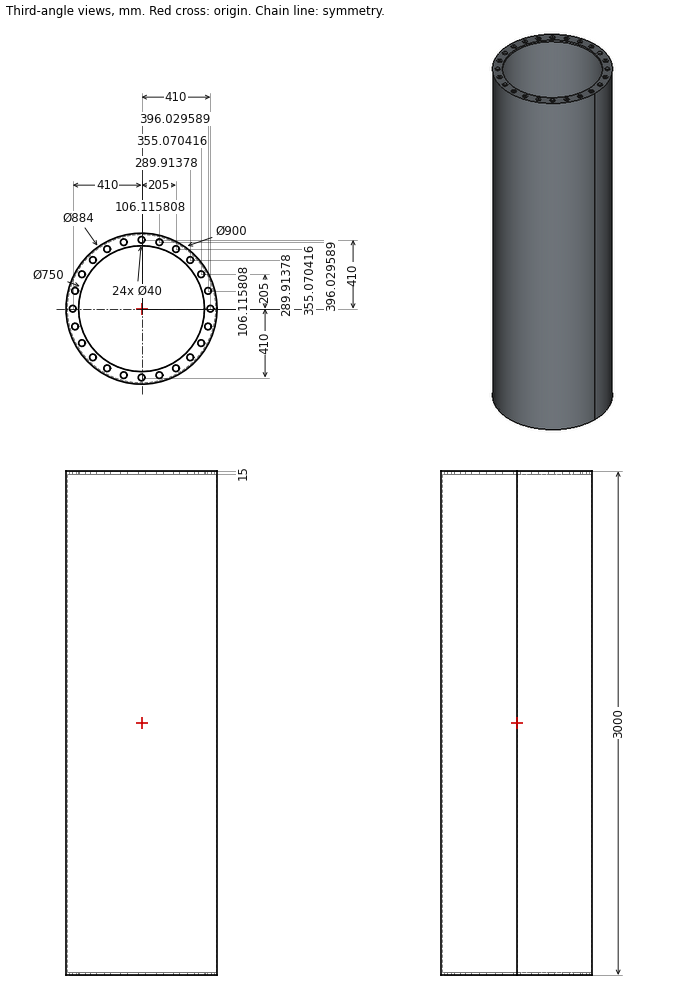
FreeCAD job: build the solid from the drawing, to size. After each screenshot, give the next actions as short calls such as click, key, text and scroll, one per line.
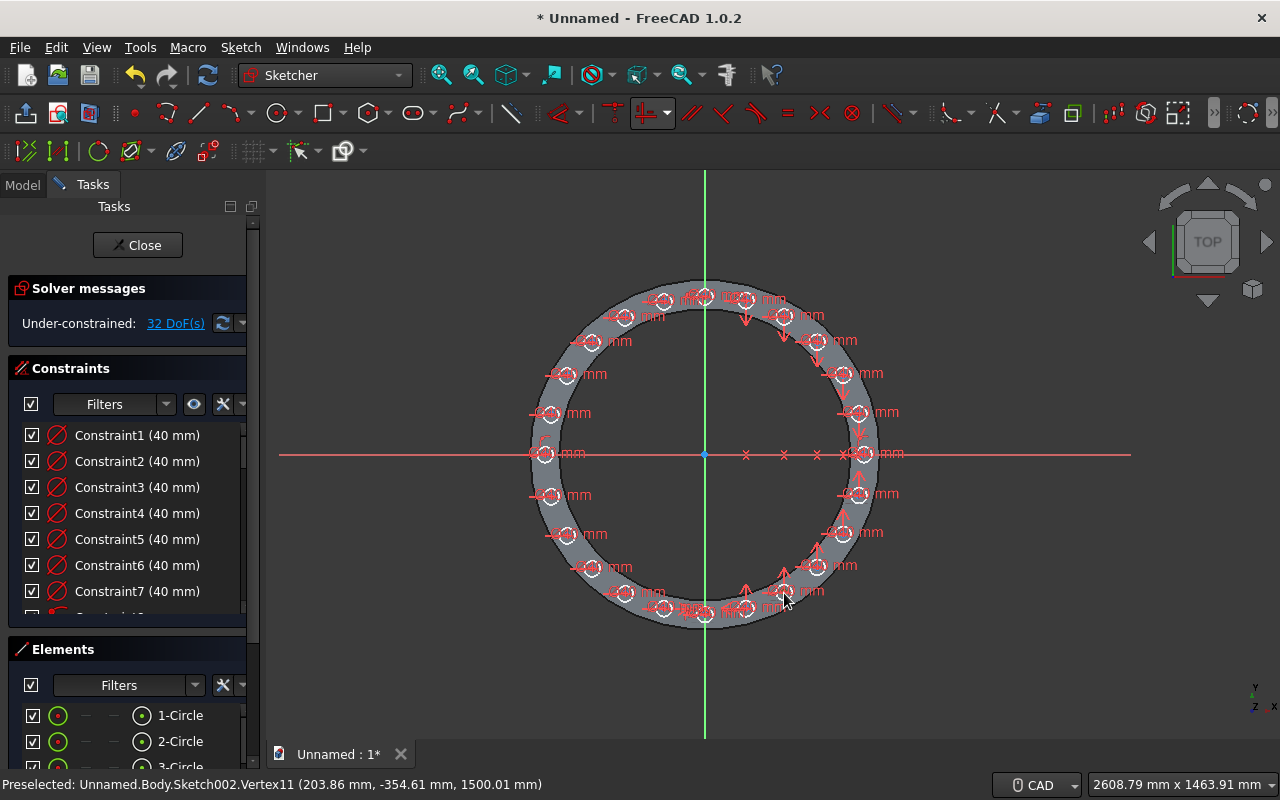
click(625, 594)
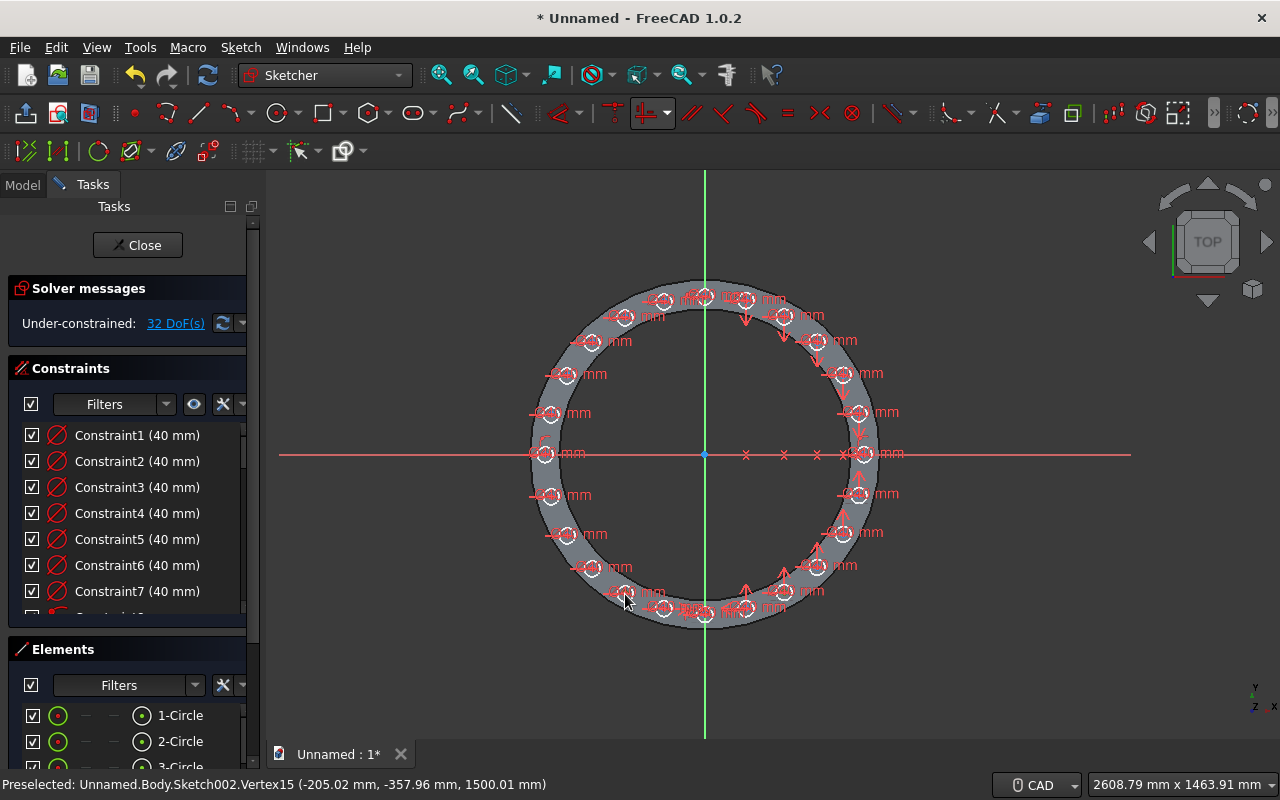
click(705, 674)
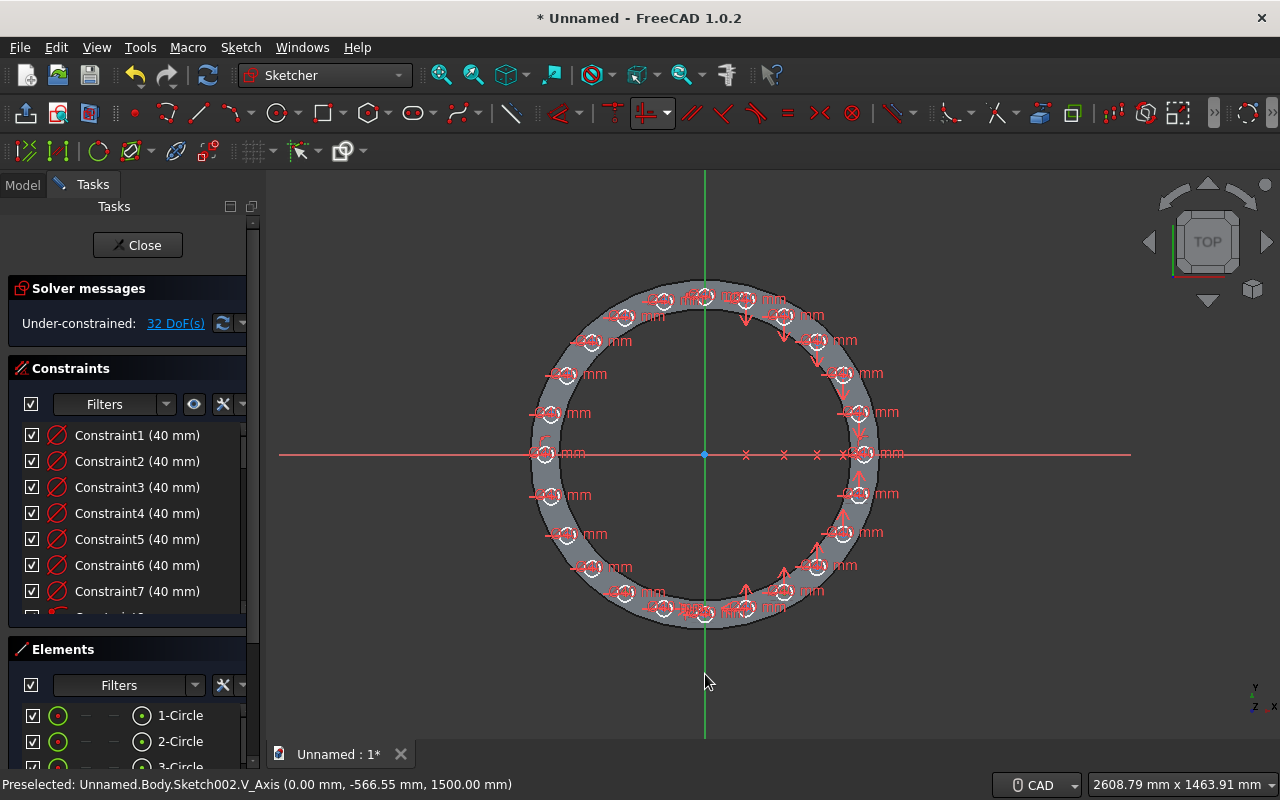
click(820, 114)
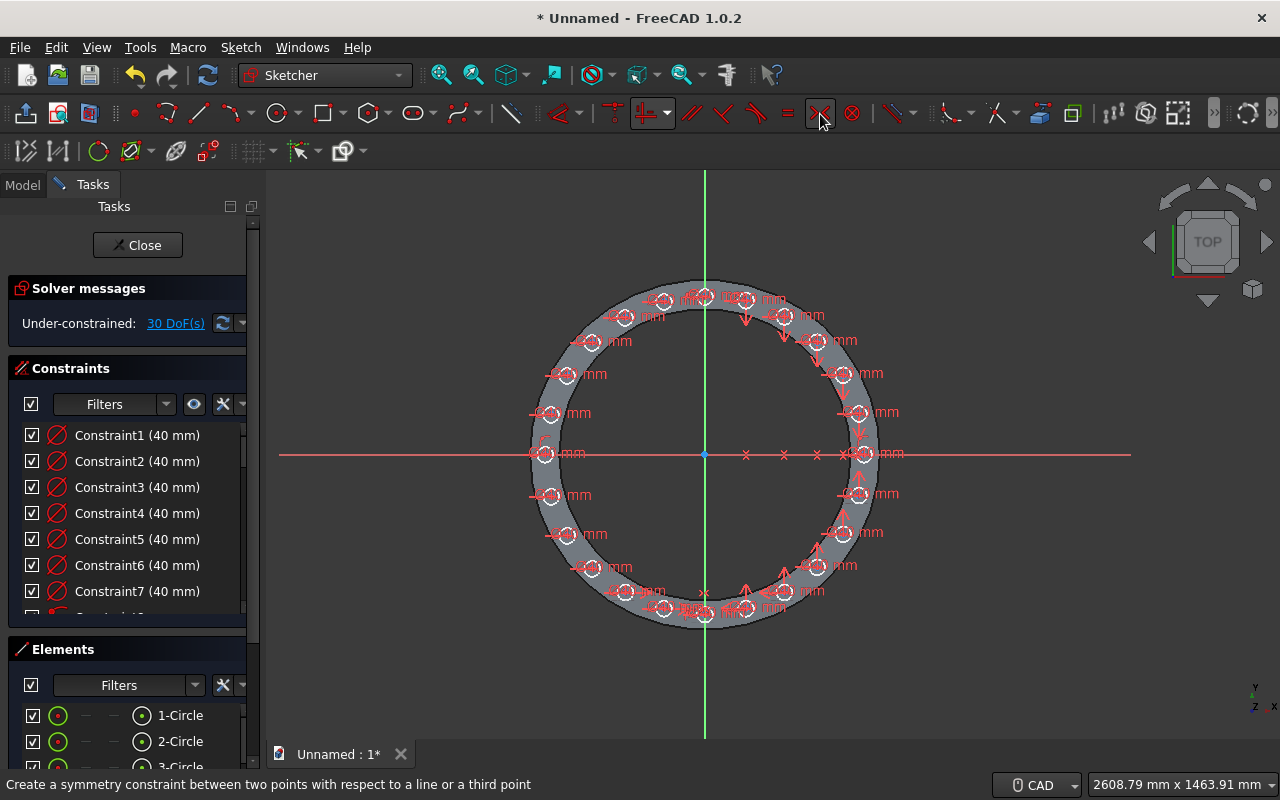
click(817, 567)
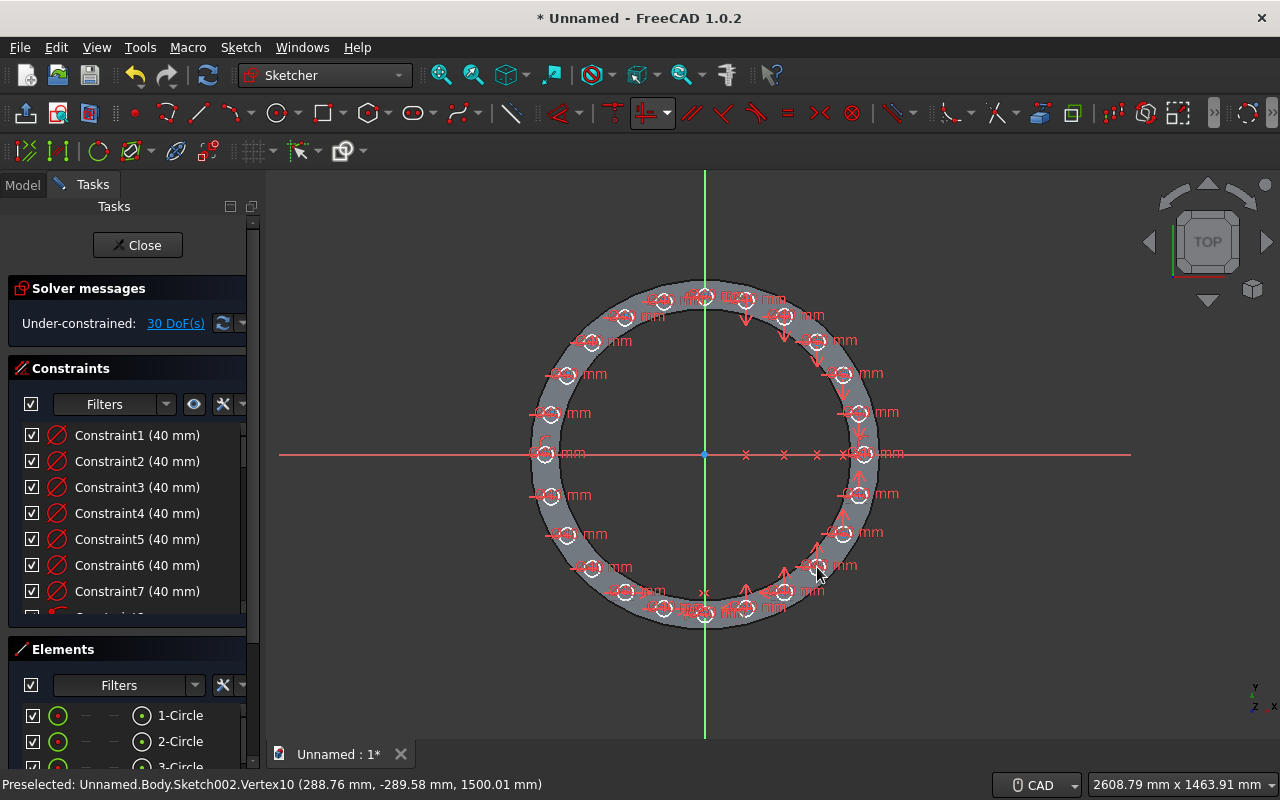
click(592, 569)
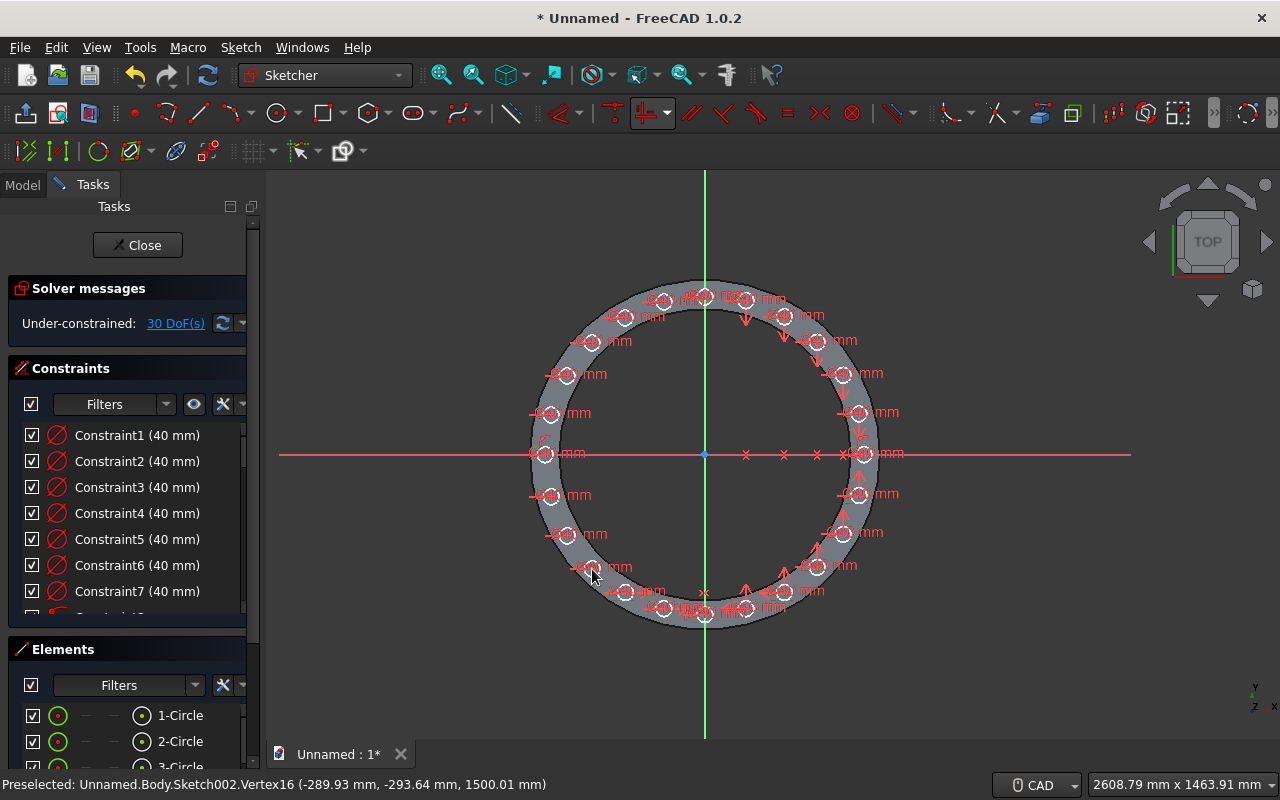
click(705, 674)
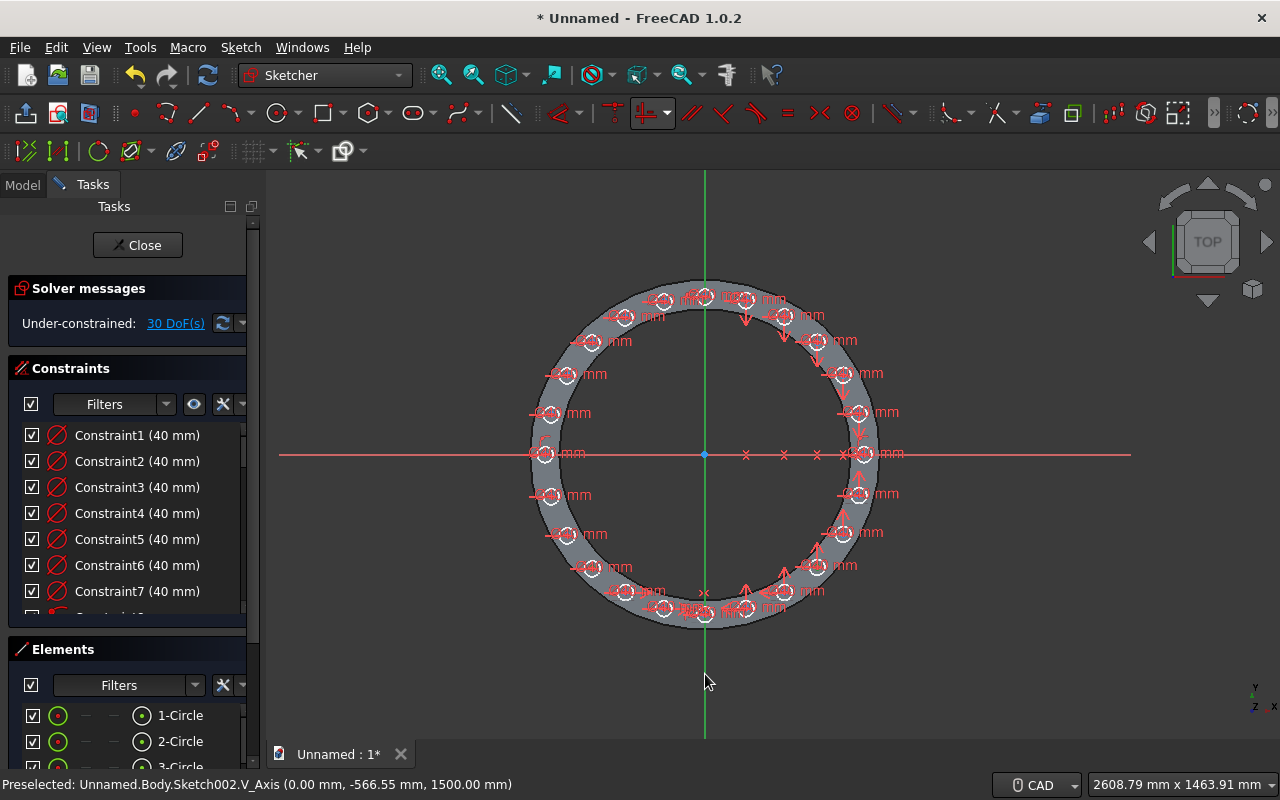
click(820, 114)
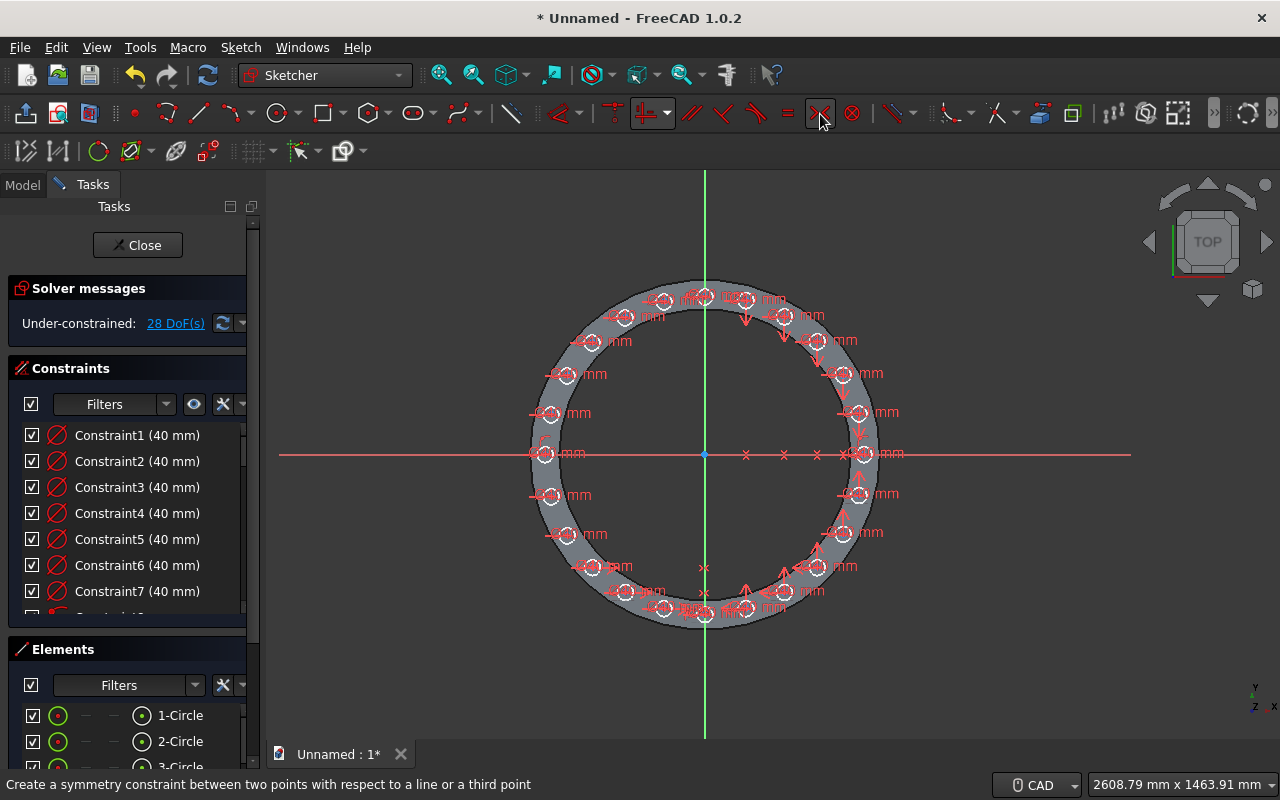
click(843, 534)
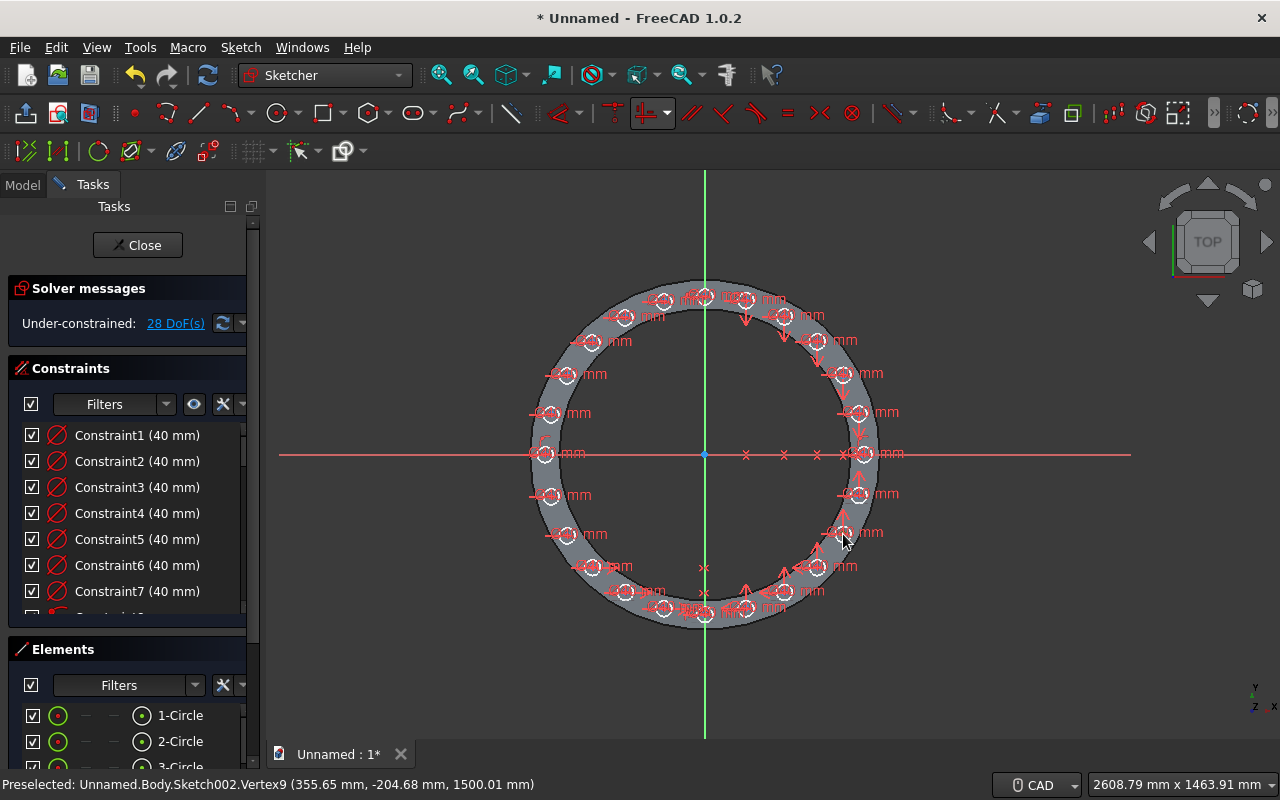
click(567, 536)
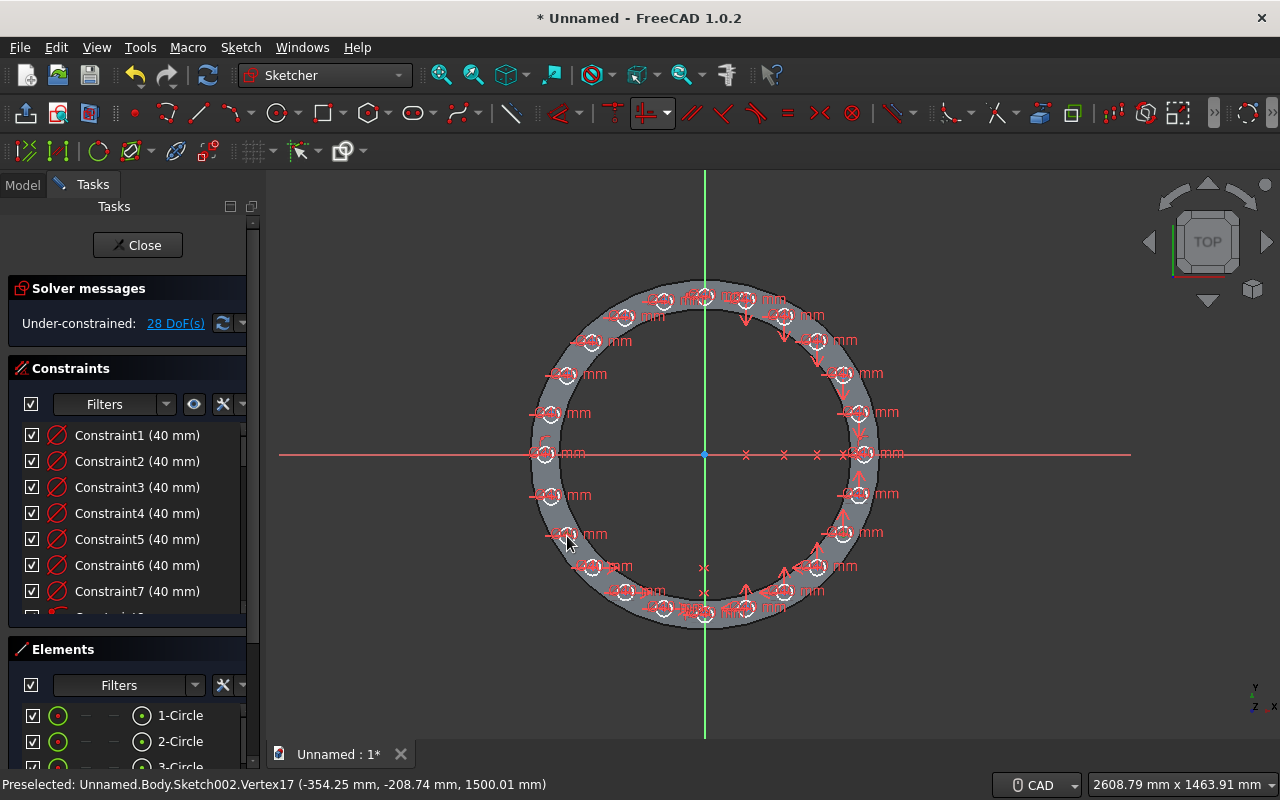
click(705, 674)